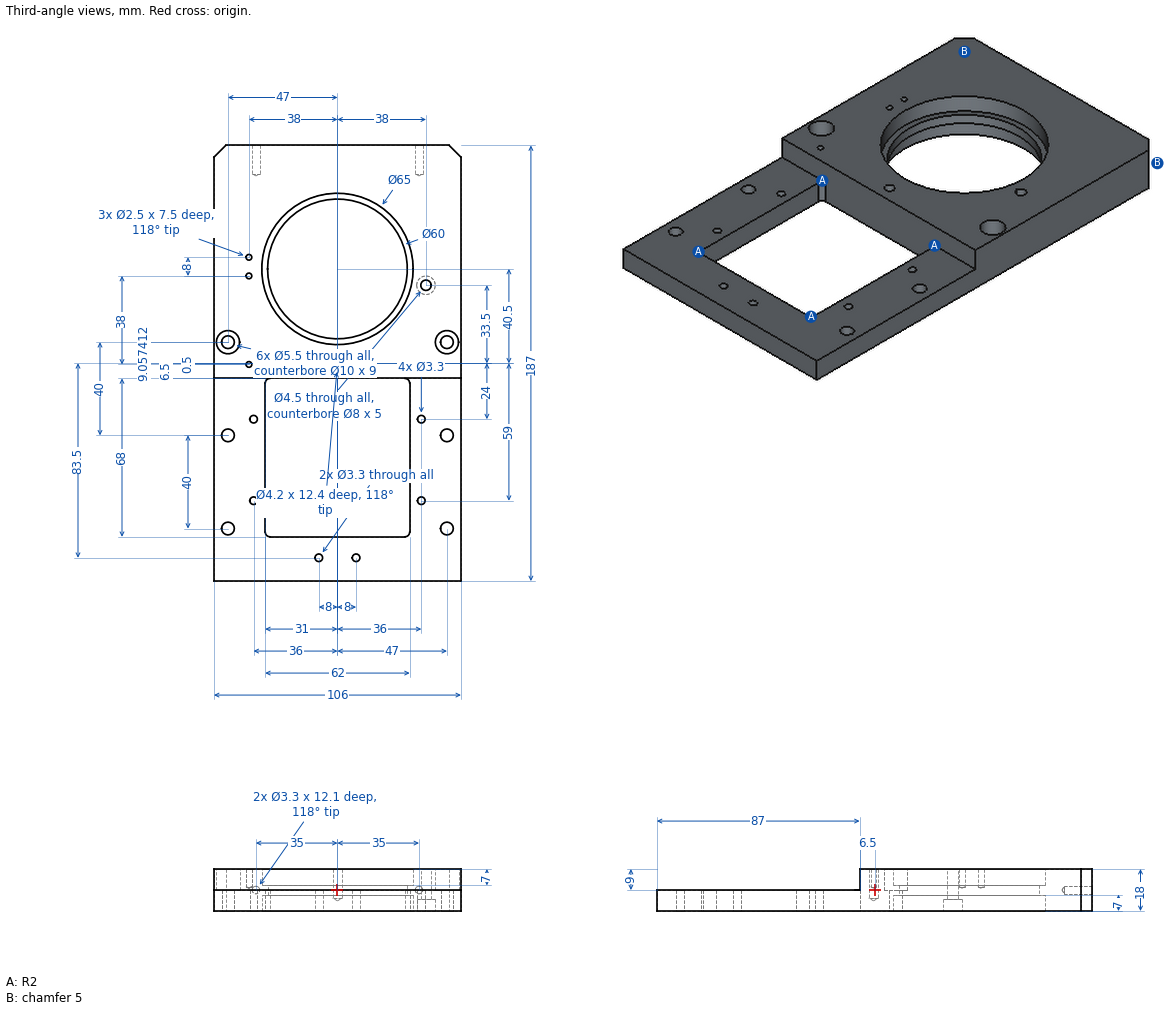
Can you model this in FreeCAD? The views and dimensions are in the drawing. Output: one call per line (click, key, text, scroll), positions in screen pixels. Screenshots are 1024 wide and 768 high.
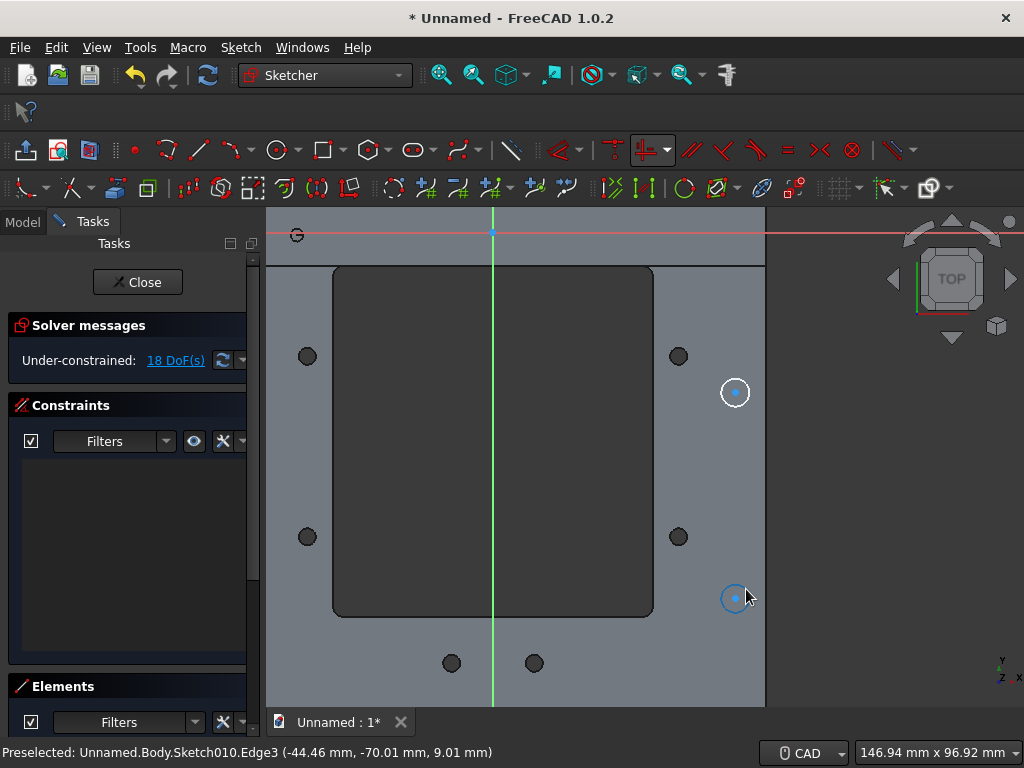
click(745, 589)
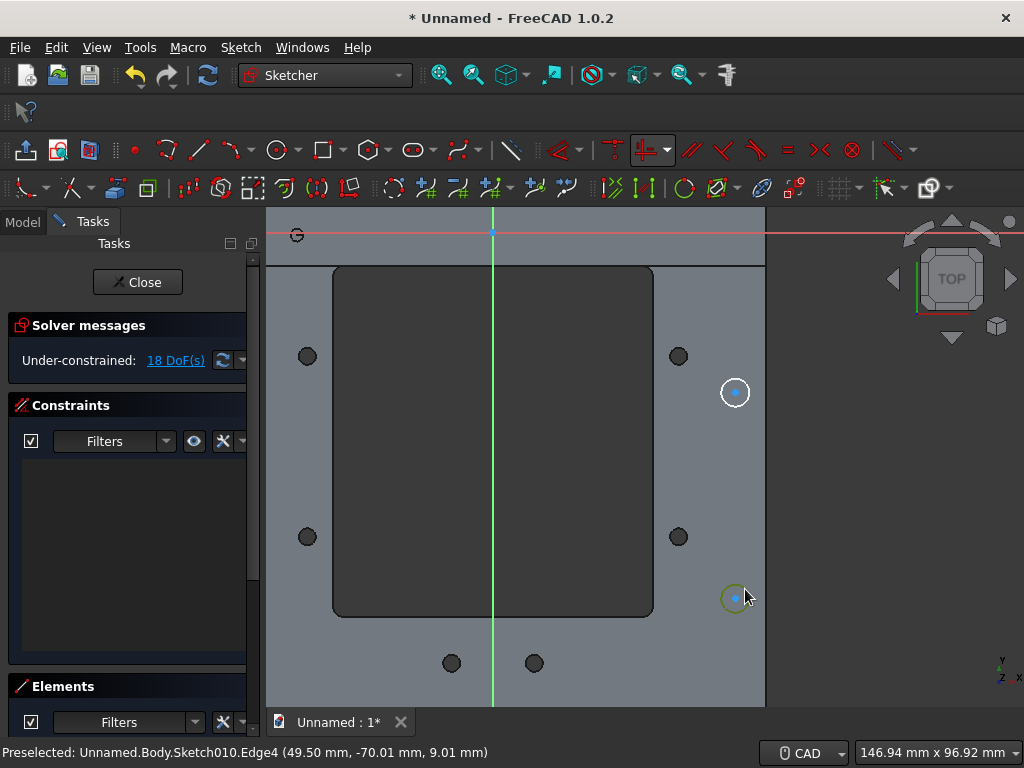
click(745, 383)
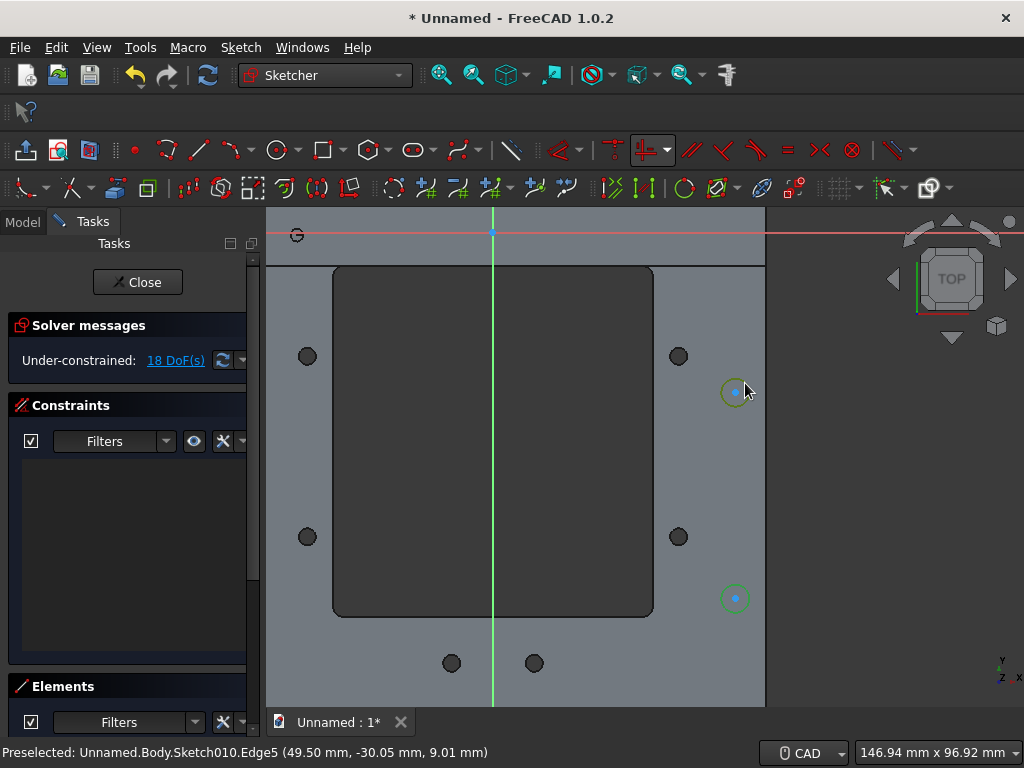
scroll(746, 589, down, 2)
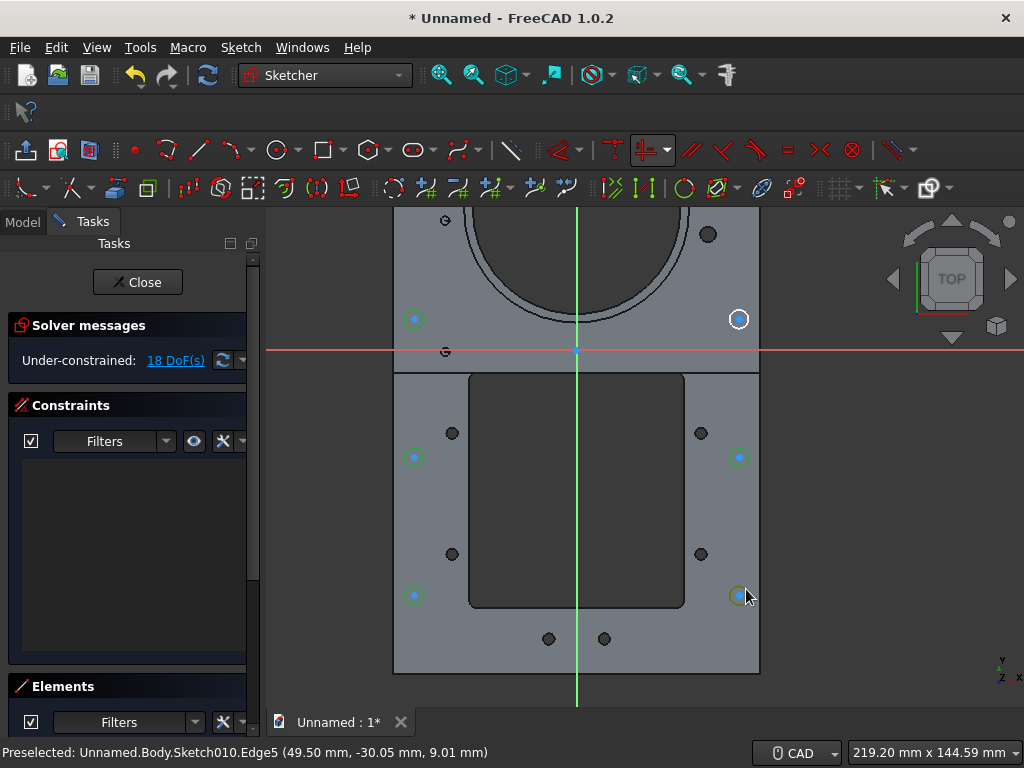
scroll(746, 313, up, 2)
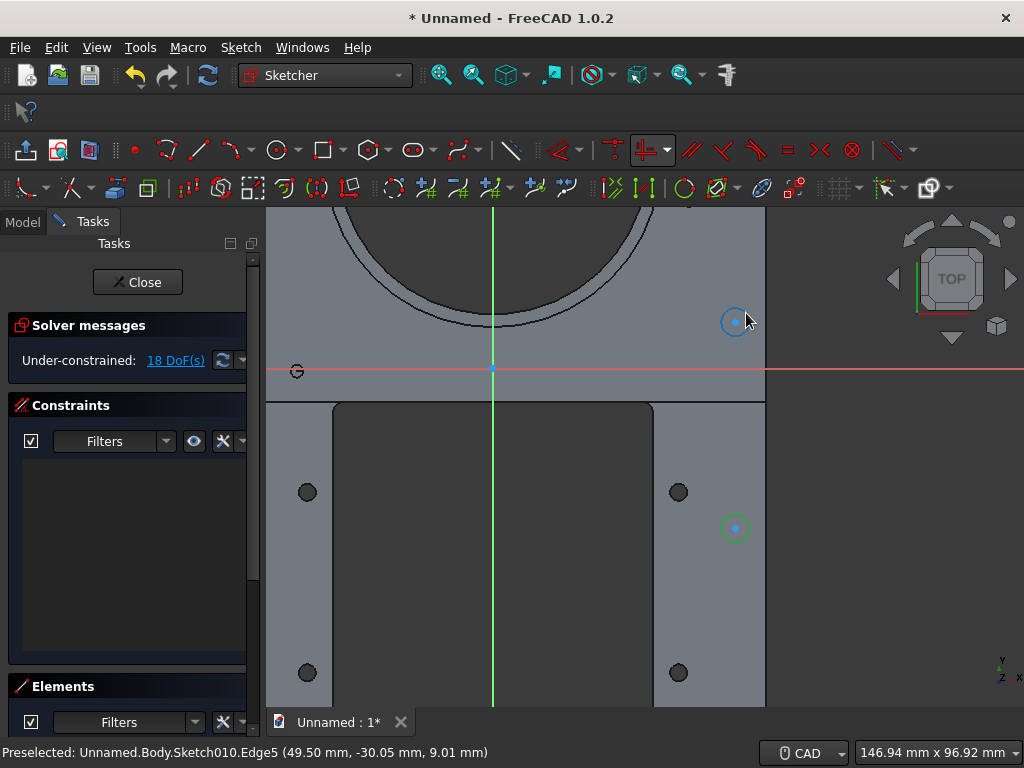
click(745, 312)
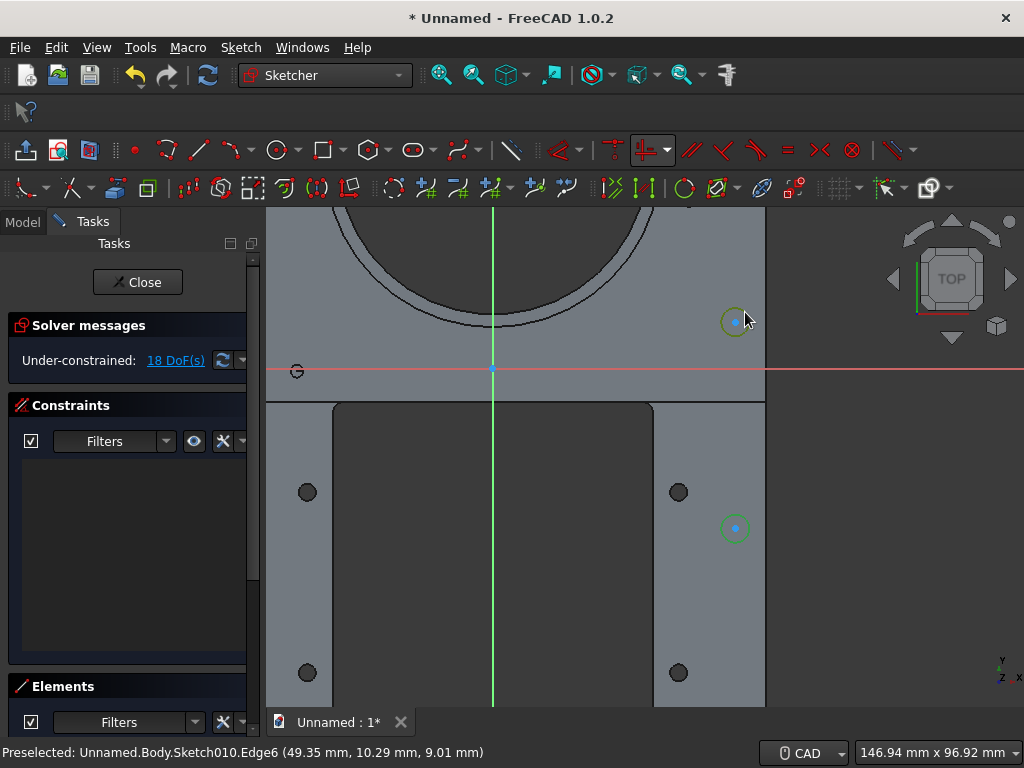
click(788, 150)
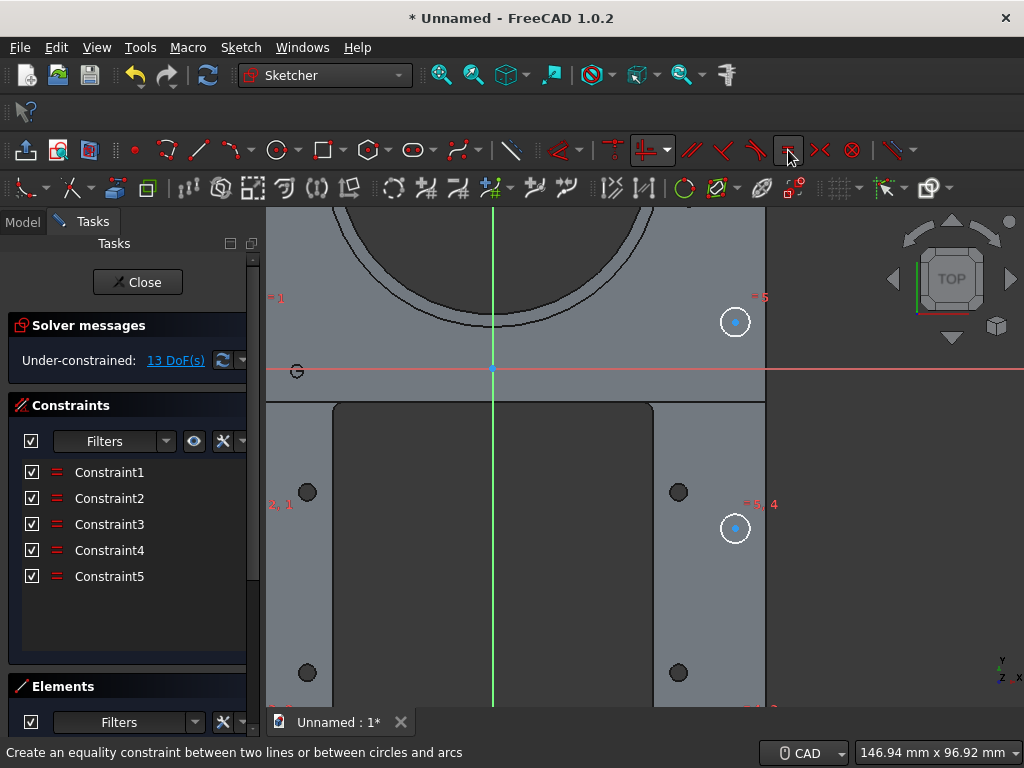
scroll(746, 312, down, 2)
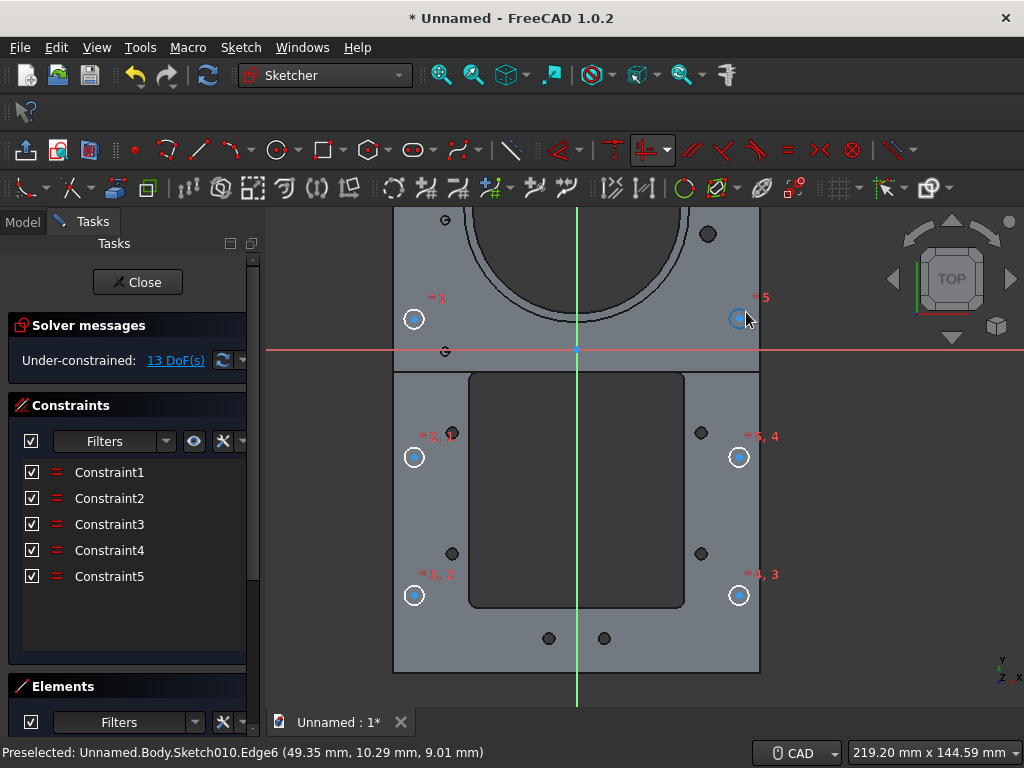
click(414, 319)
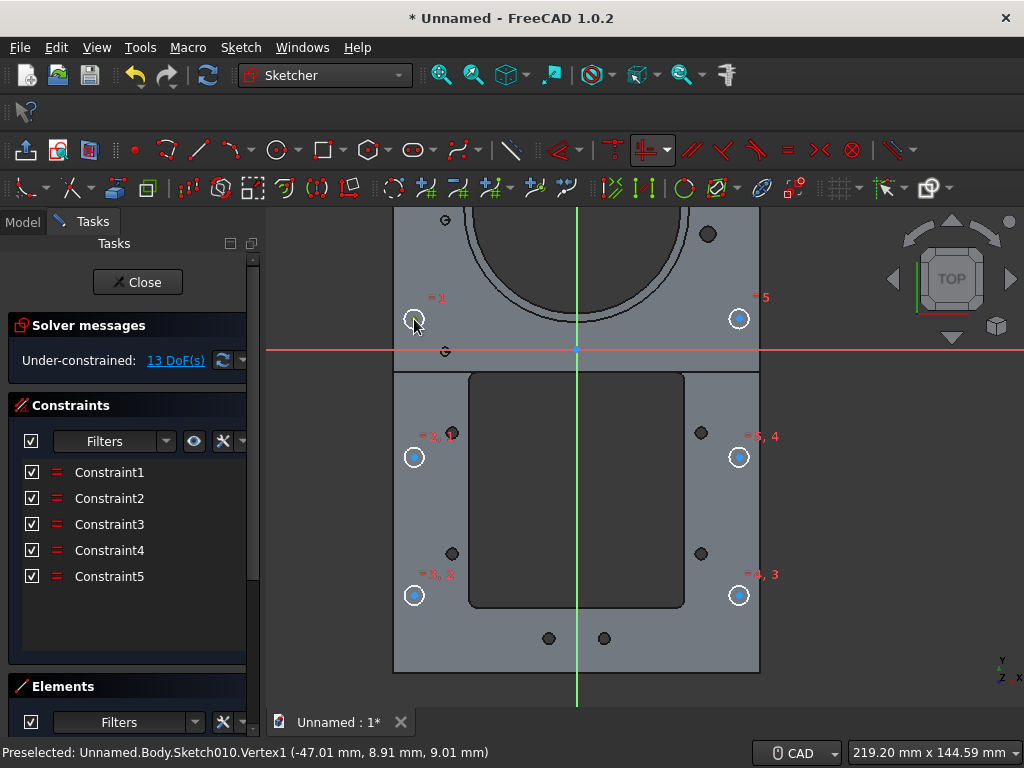
click(414, 457)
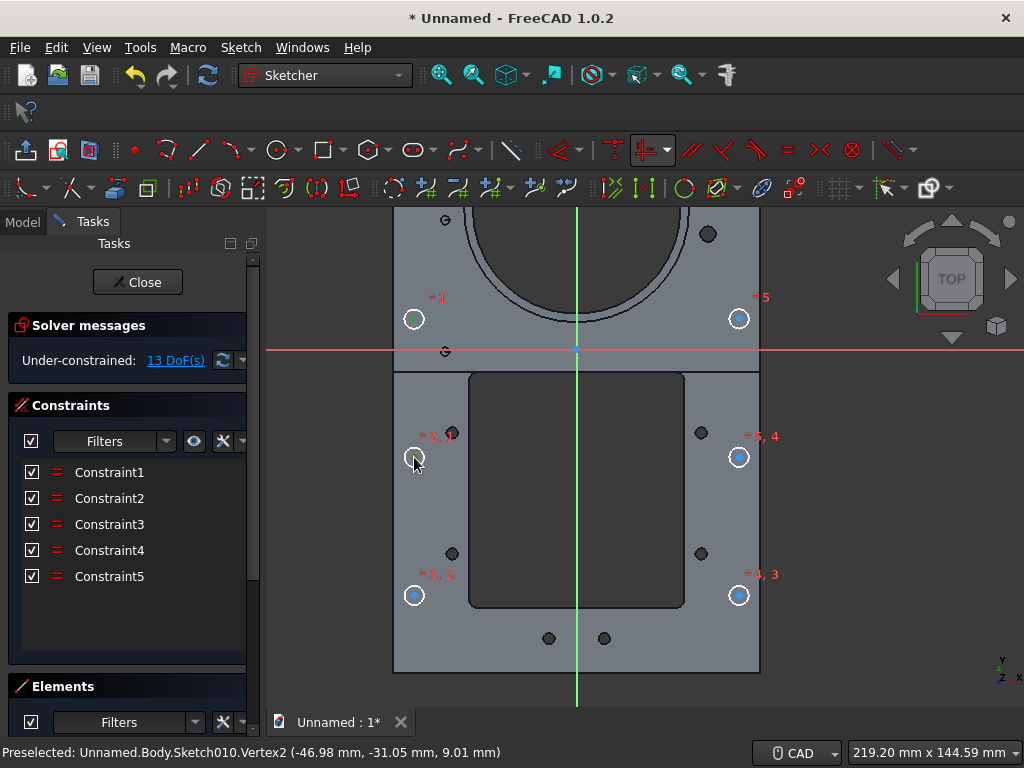
click(670, 150)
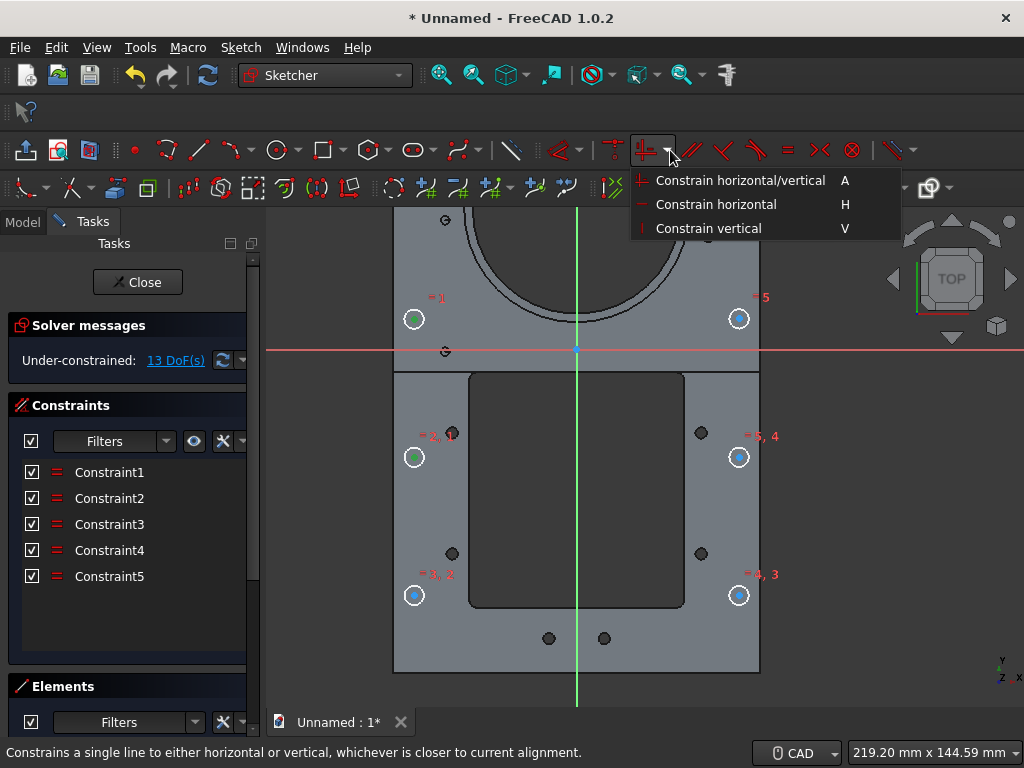
click(766, 228)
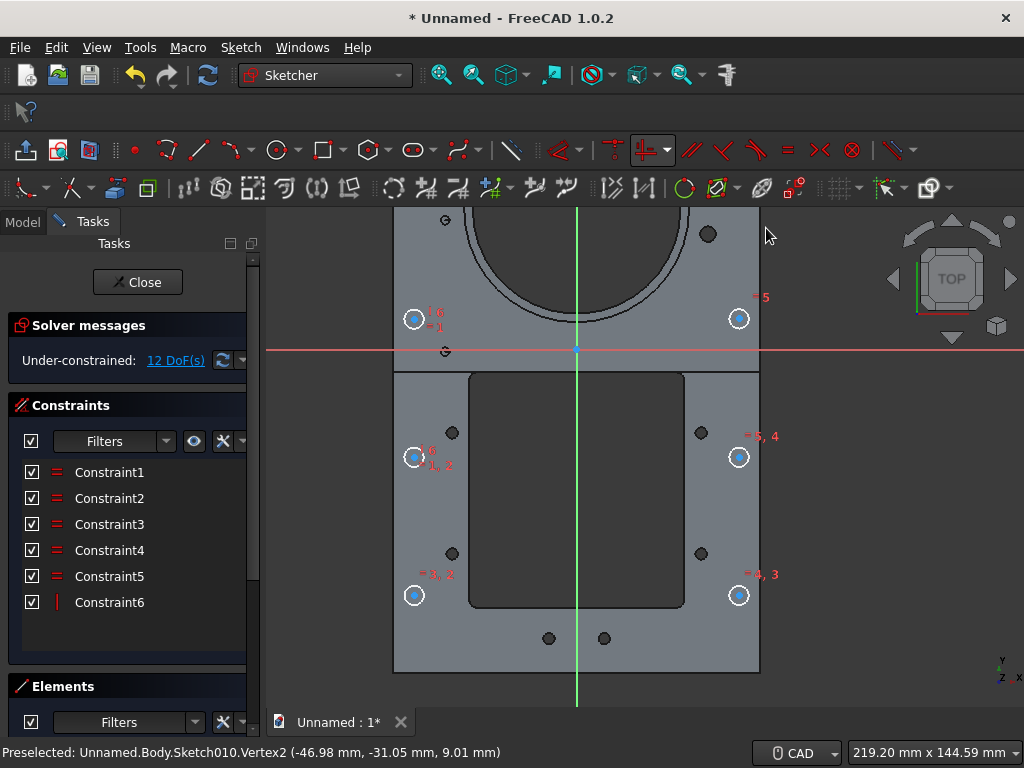
click(414, 457)